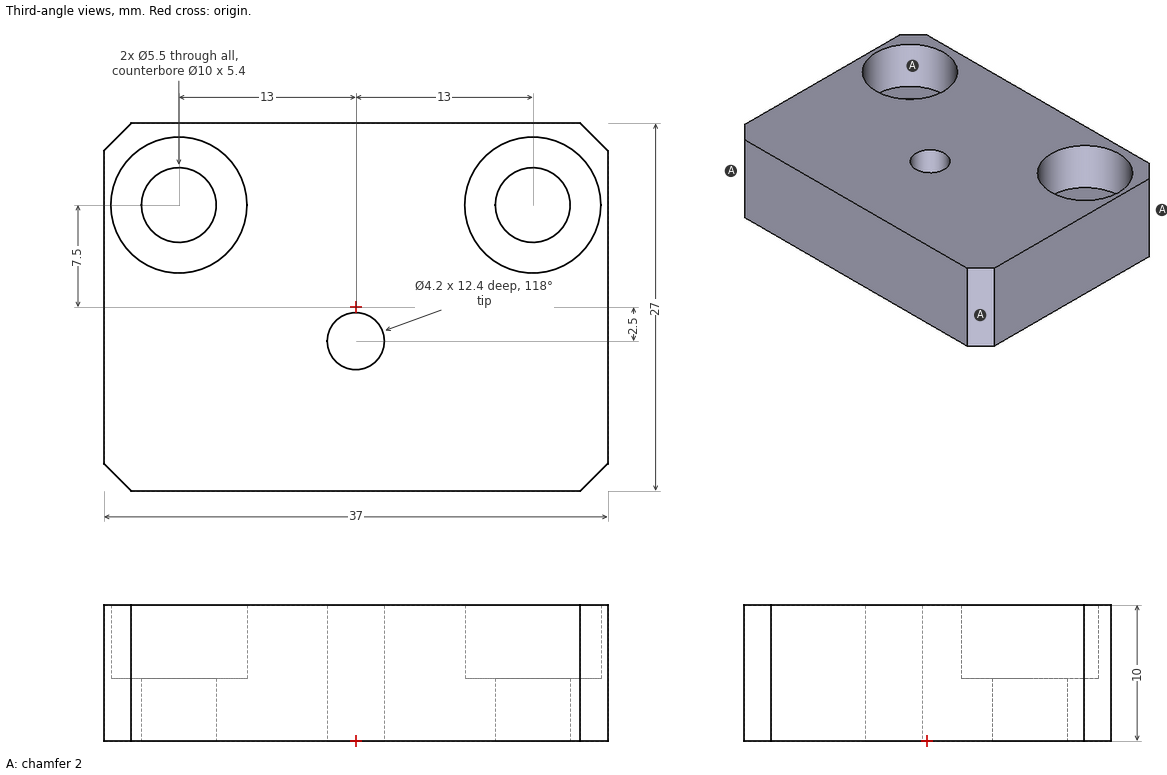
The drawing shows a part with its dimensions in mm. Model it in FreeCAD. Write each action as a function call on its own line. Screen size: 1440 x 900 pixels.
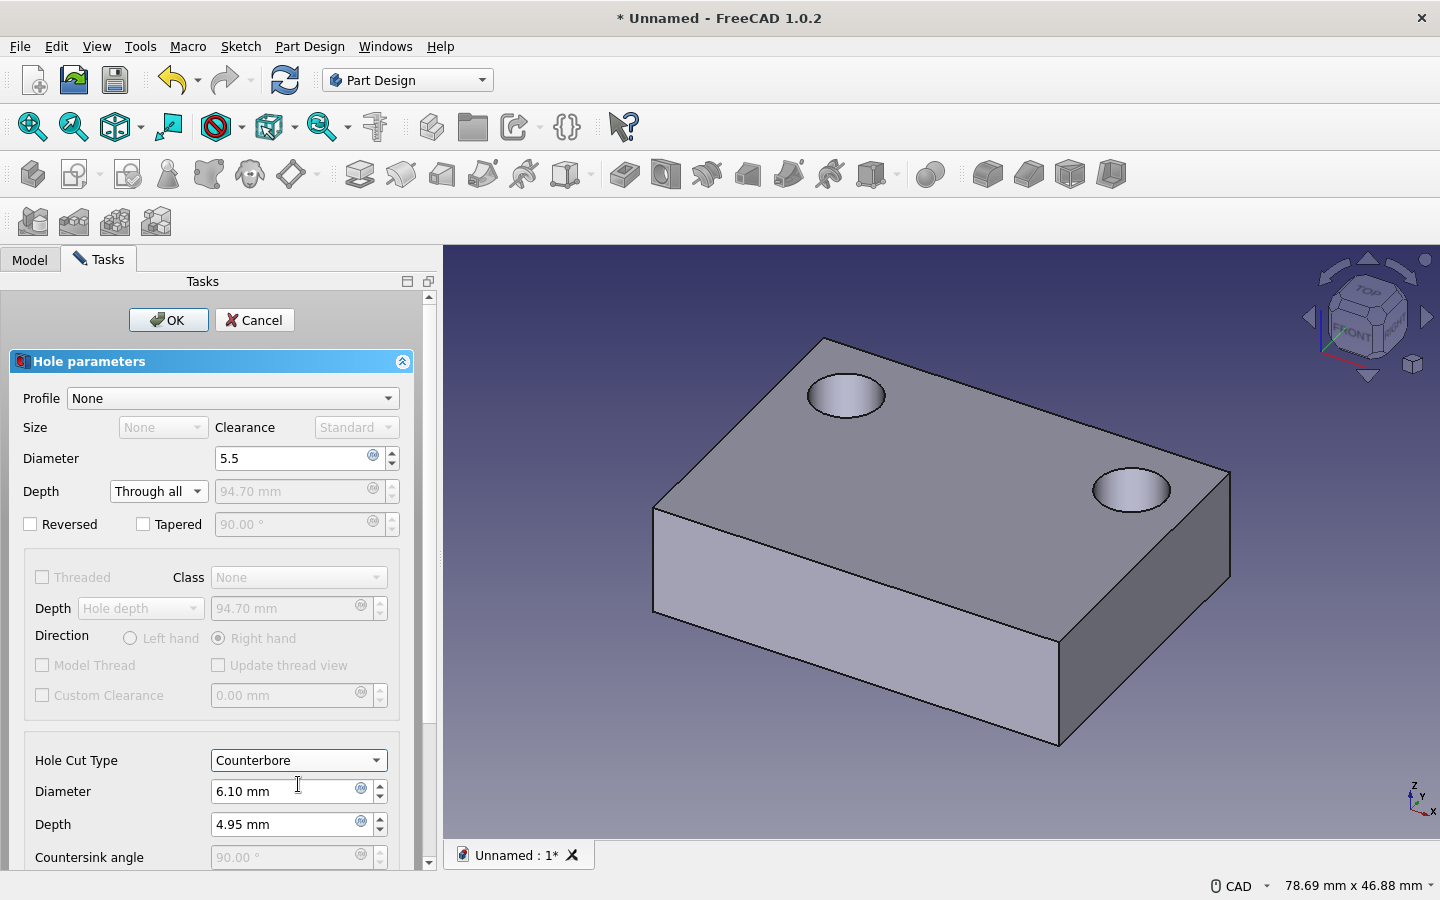
triple_click(292, 792)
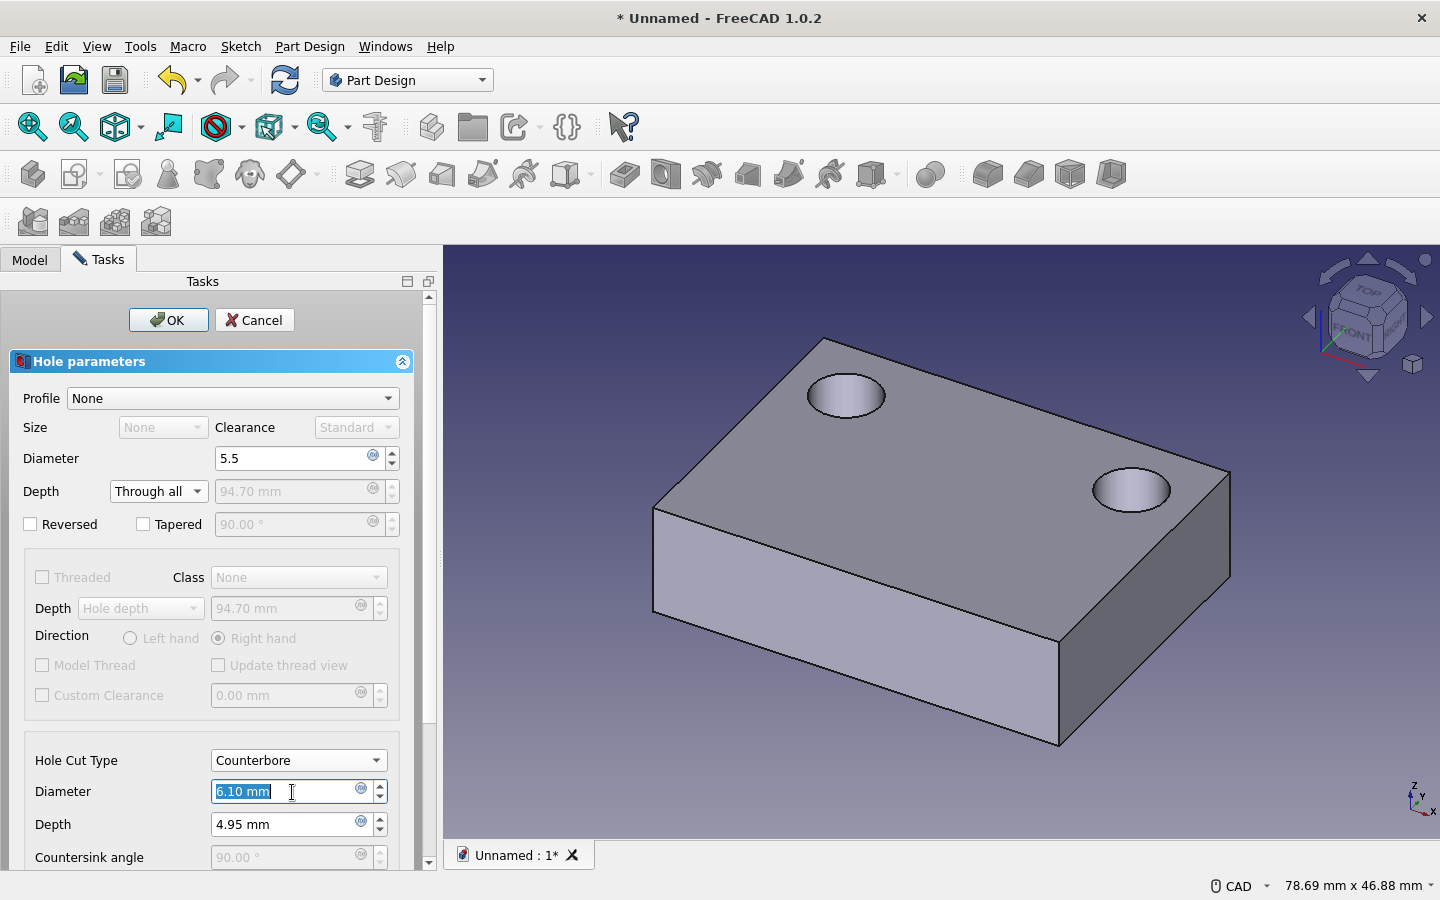
text(10)
key(Tab)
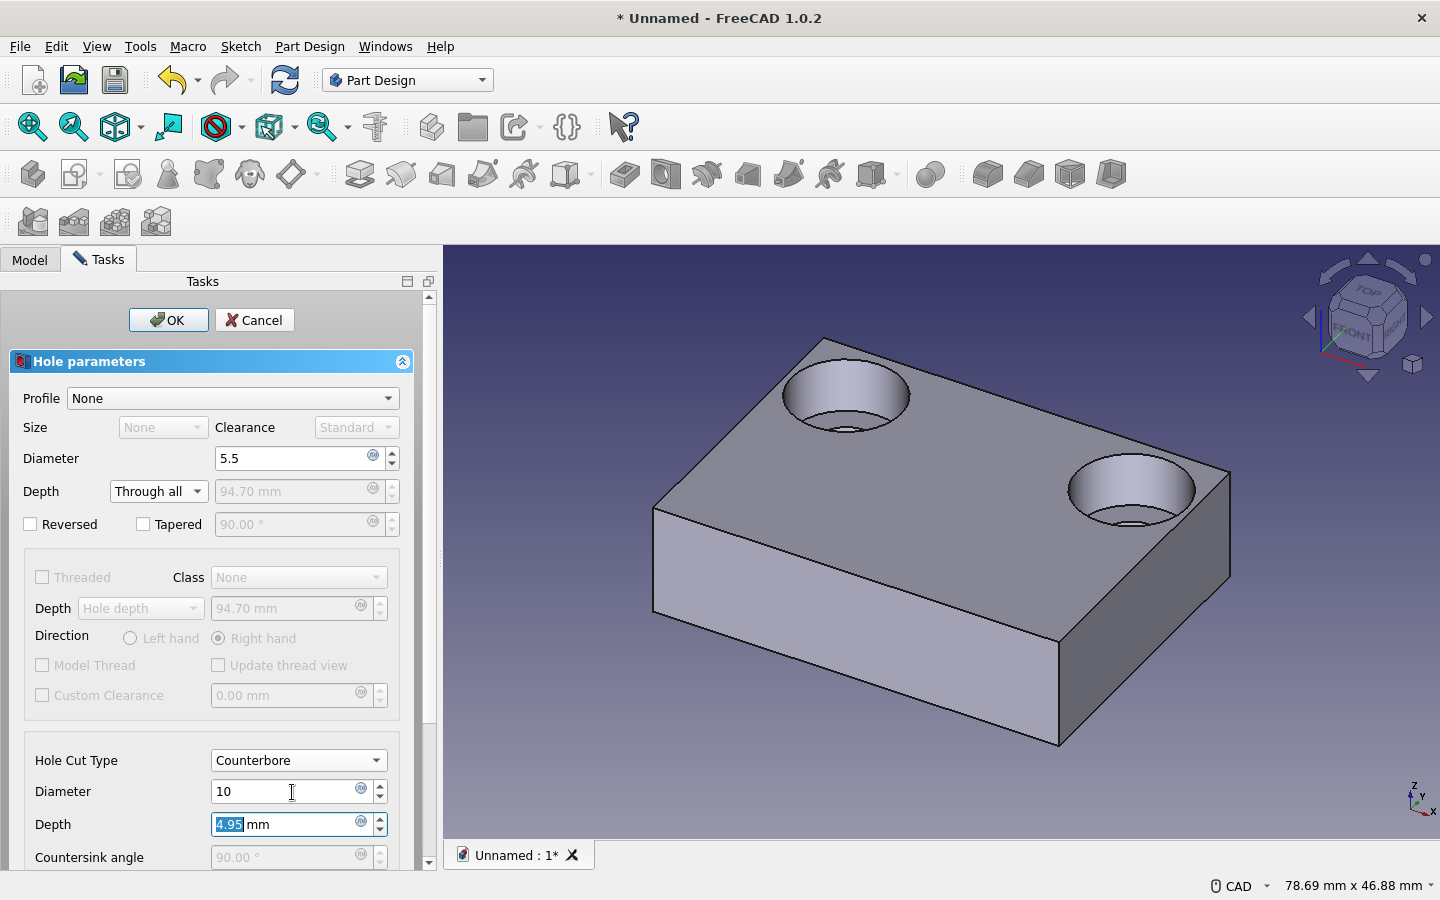
text(5.4)
key(Tab)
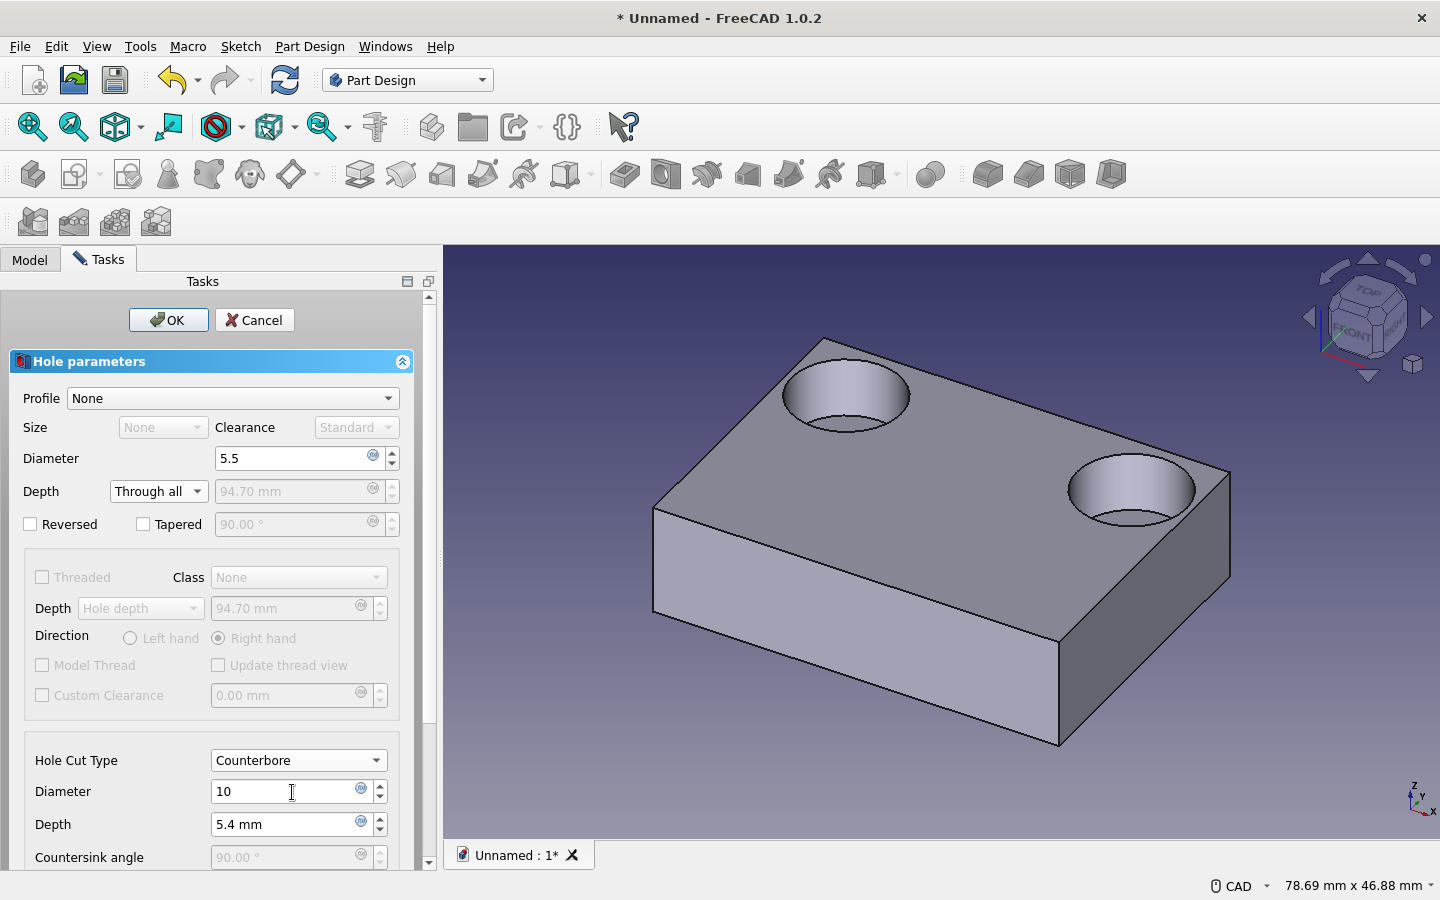
click(169, 320)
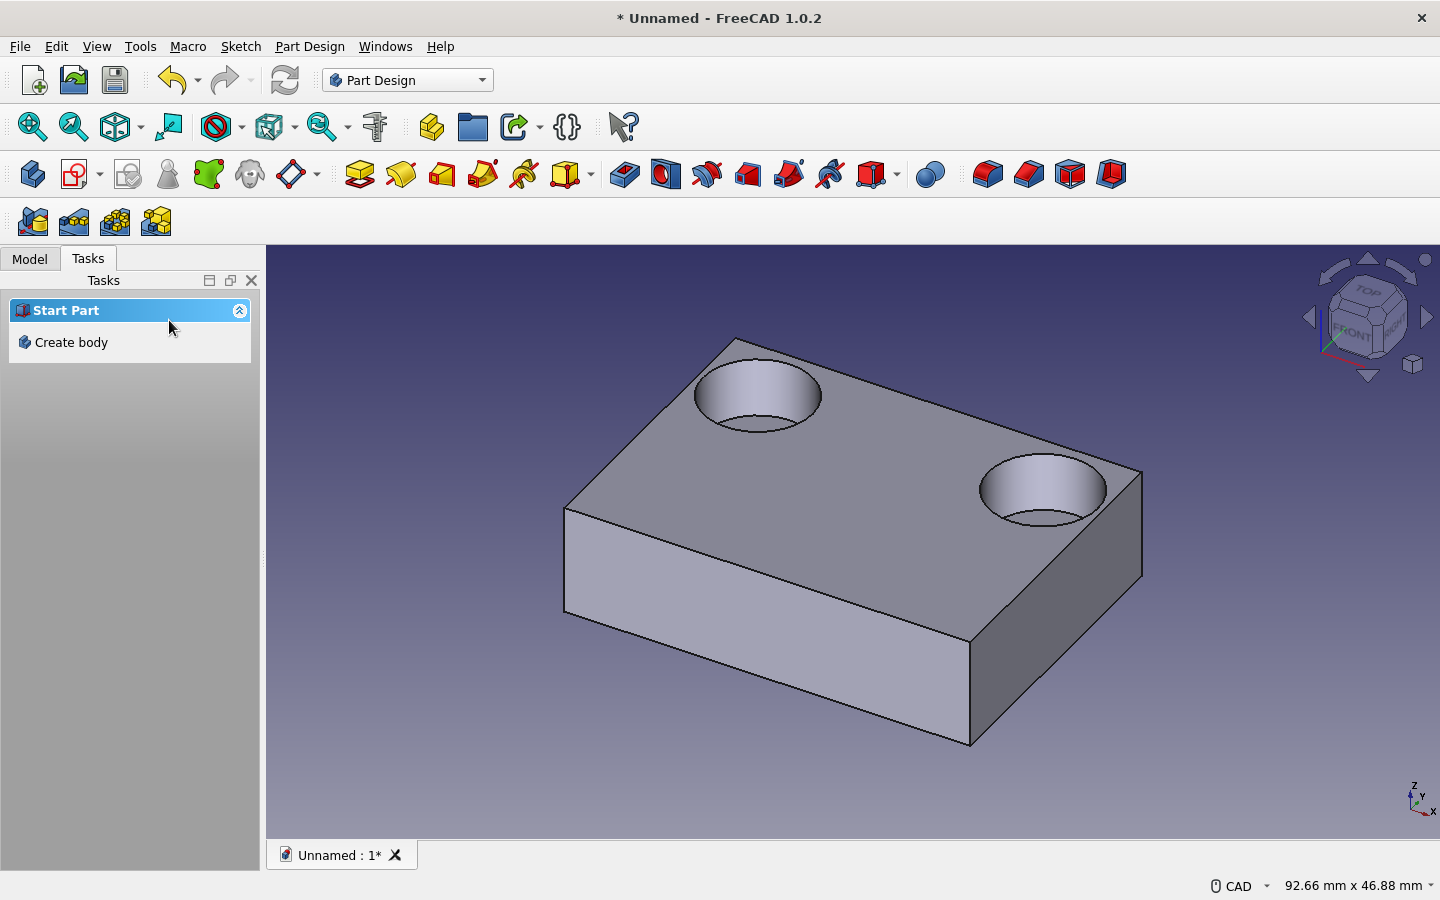
click(853, 489)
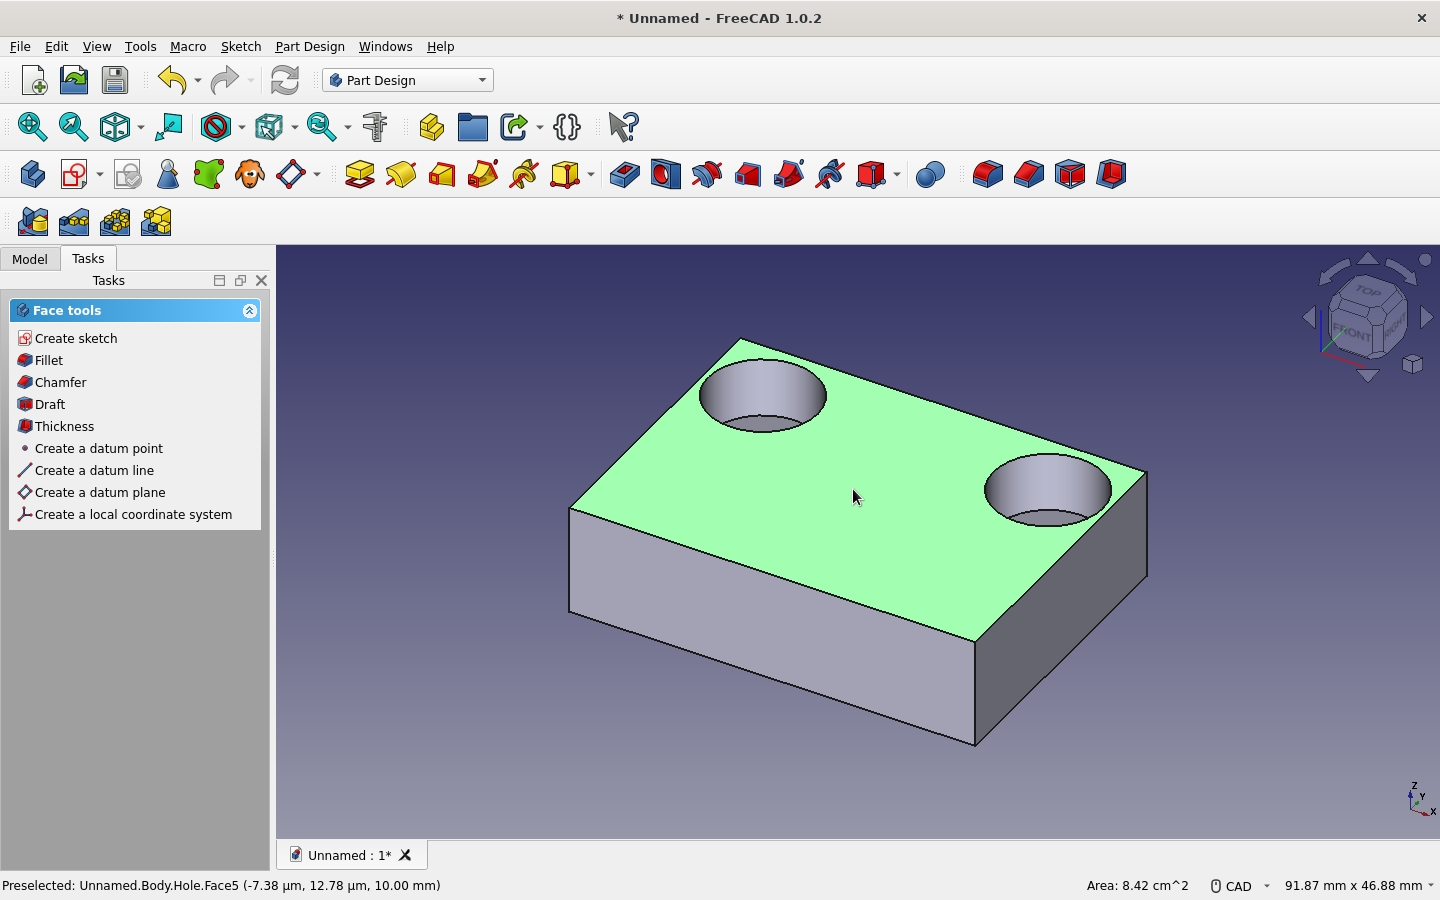
click(74, 174)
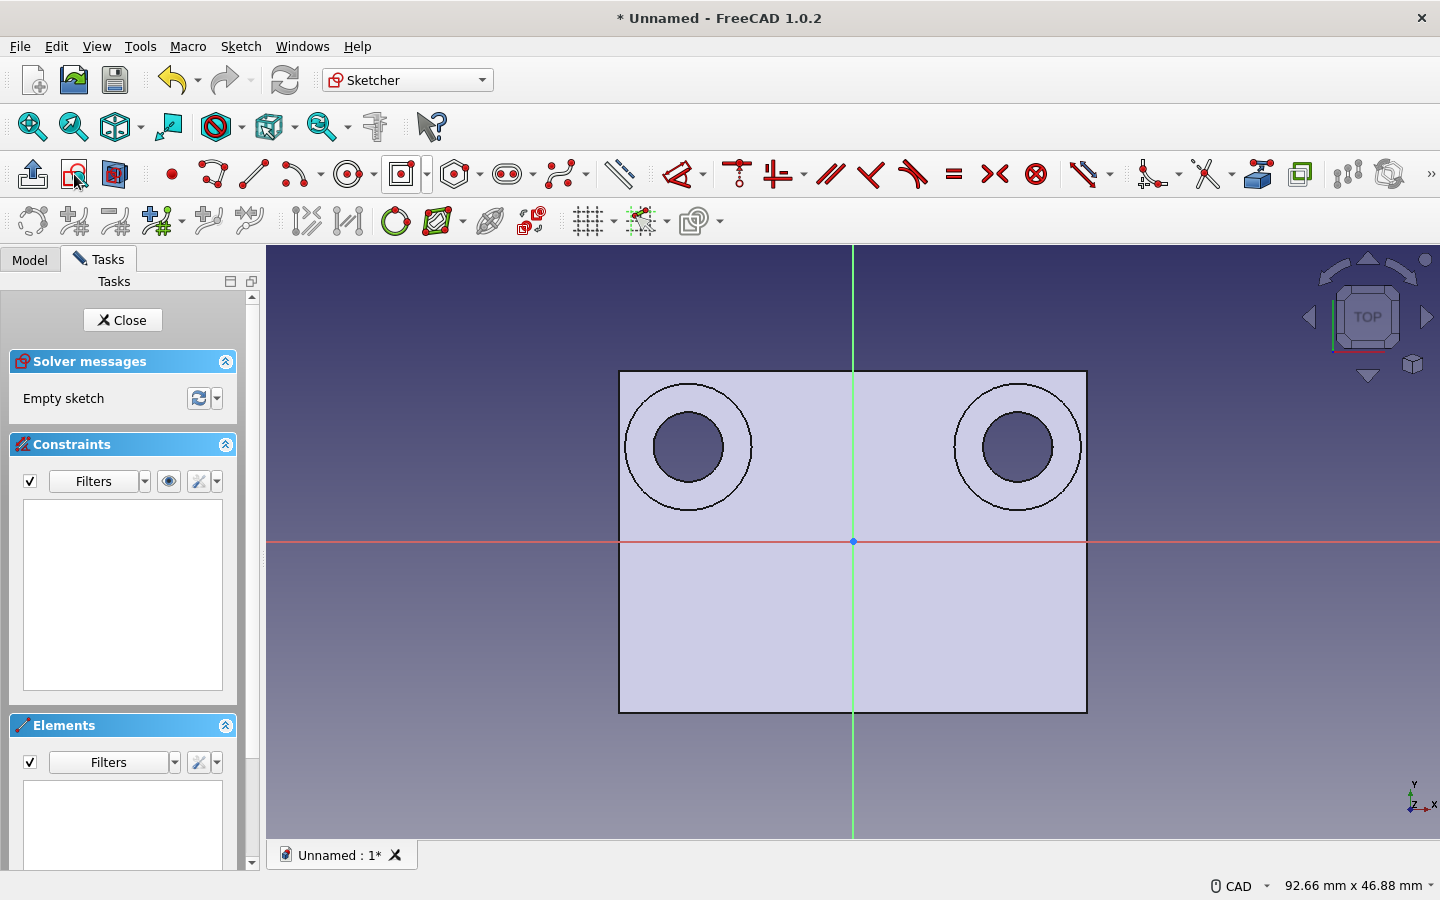
scroll(867, 577, up, 9)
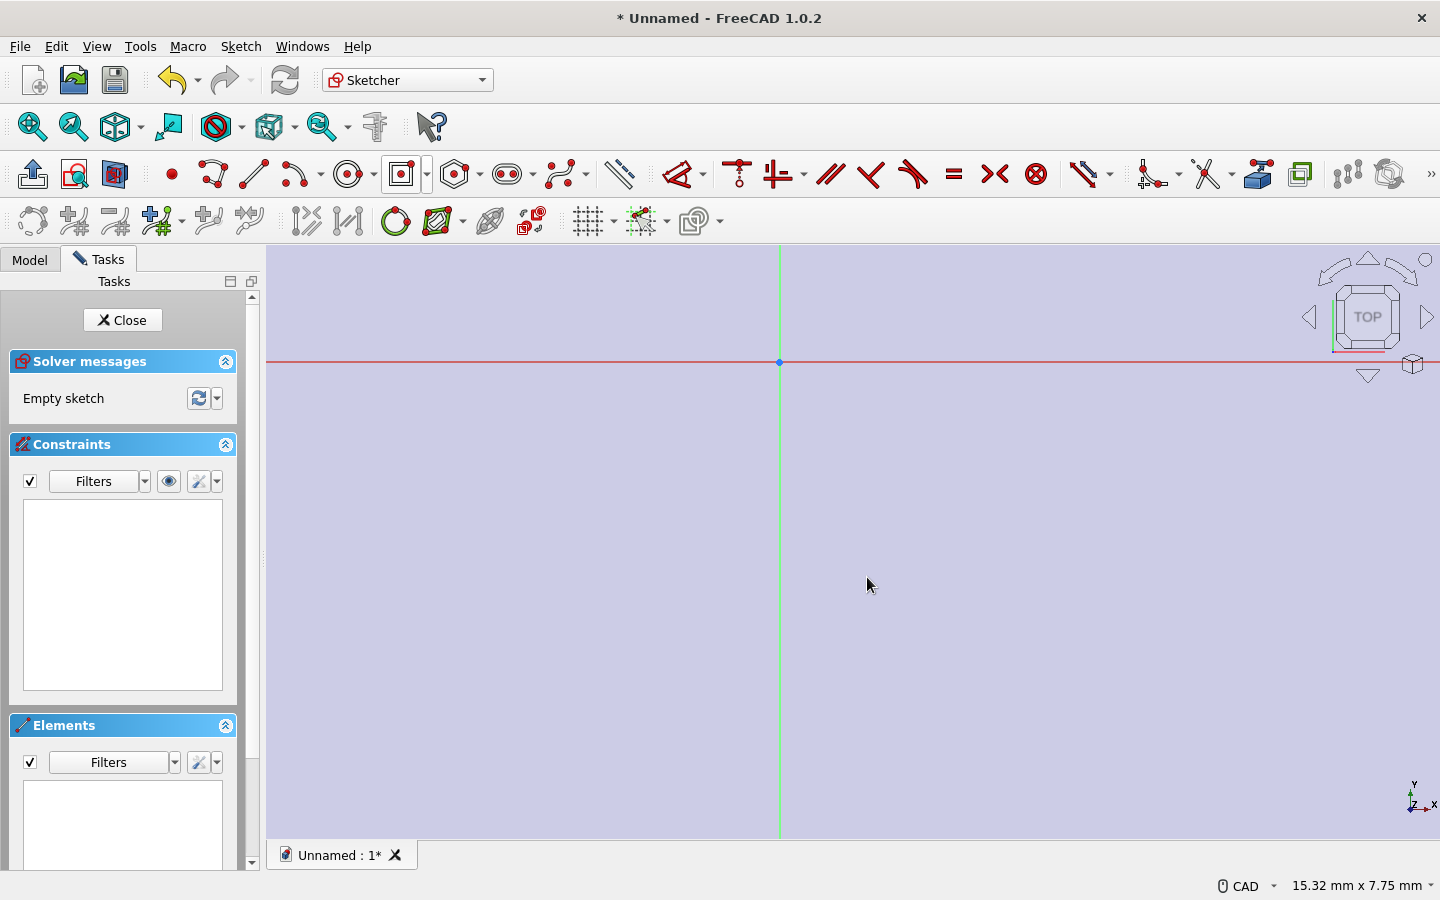
click(348, 174)